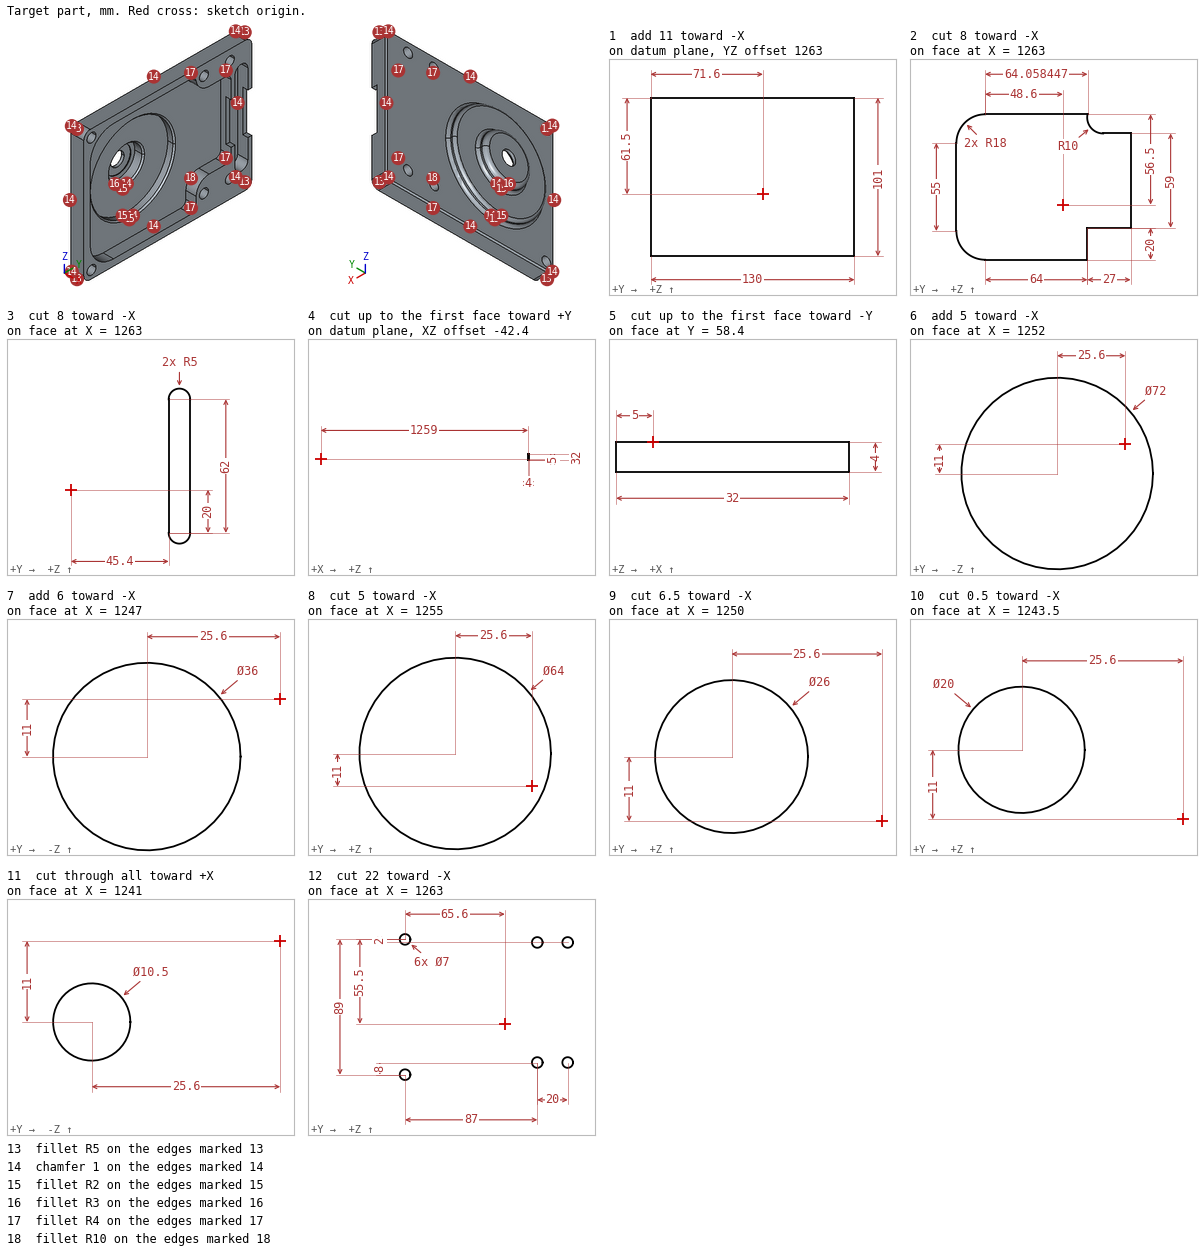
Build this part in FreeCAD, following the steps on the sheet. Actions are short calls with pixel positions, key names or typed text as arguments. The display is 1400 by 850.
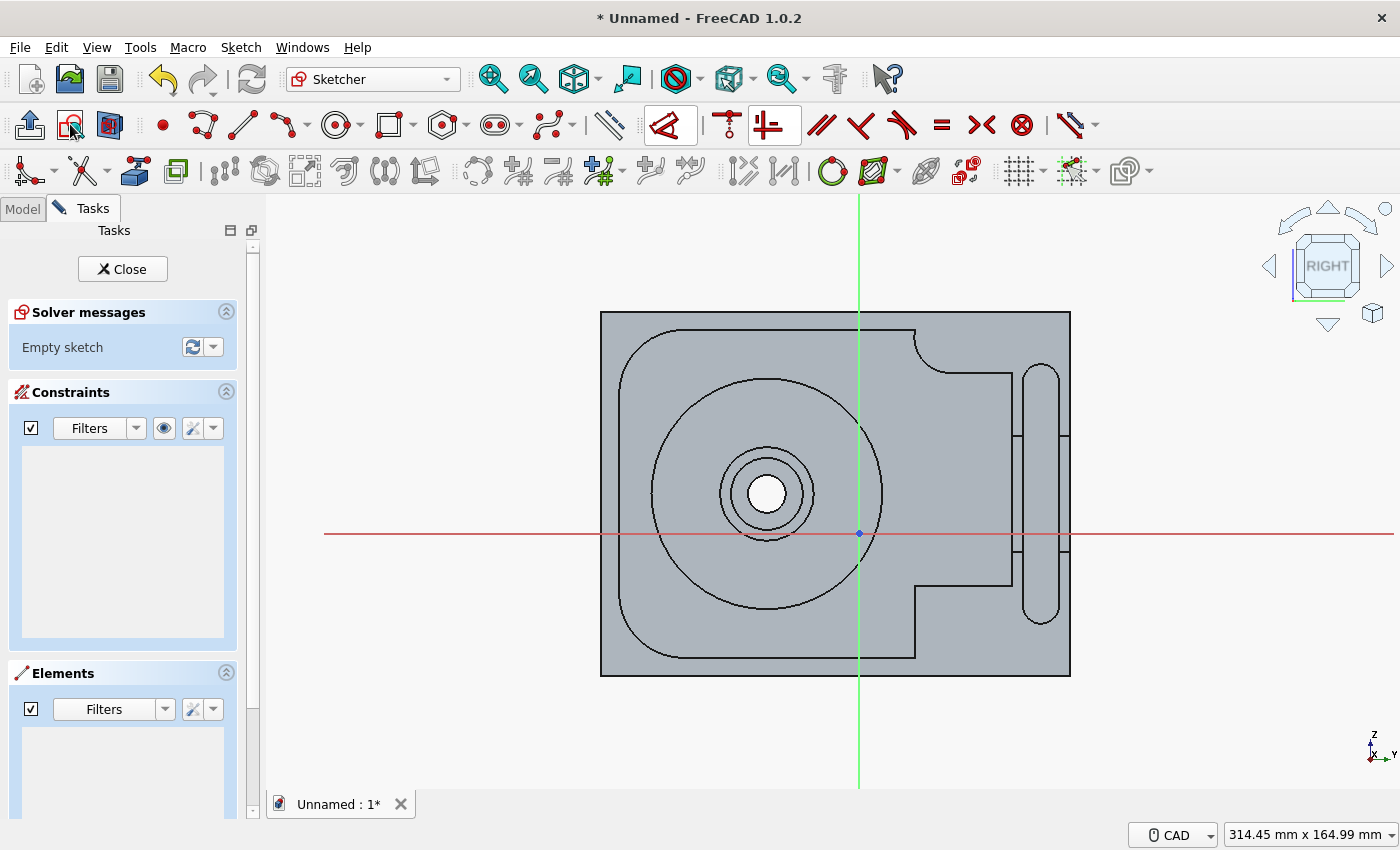
key(g)
key(c)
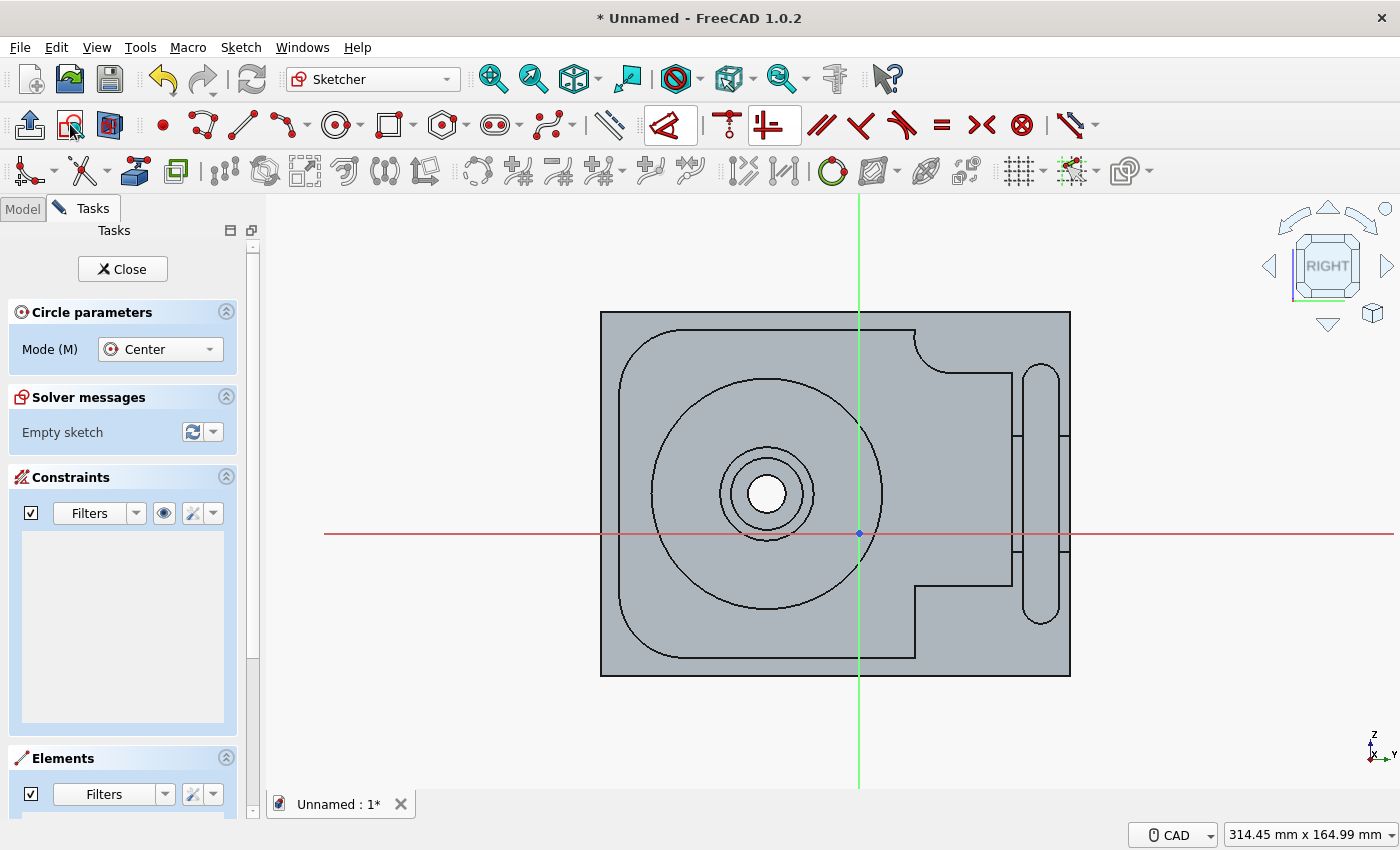
scroll(623, 333, up, 3)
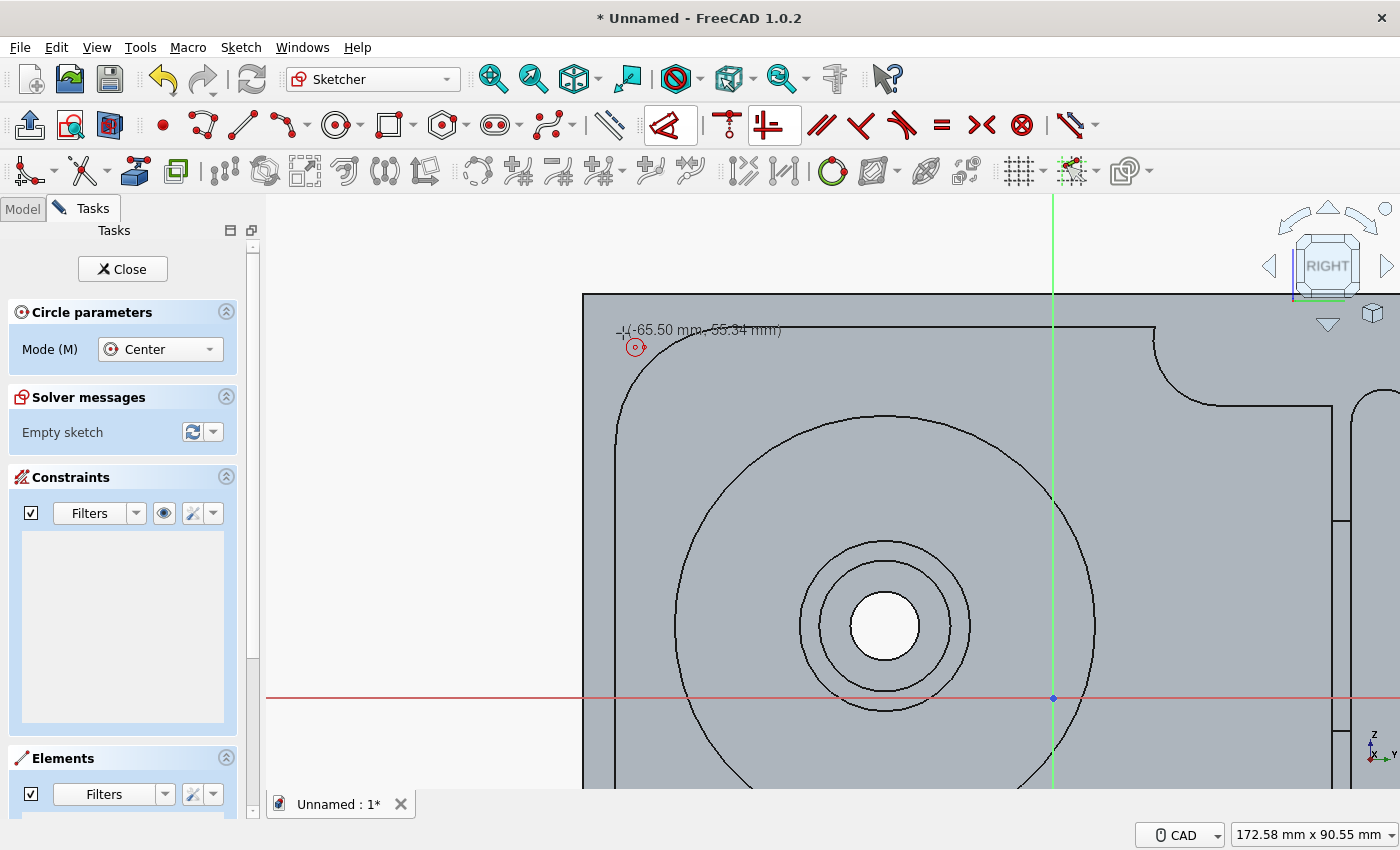
click(622, 334)
move(638, 317)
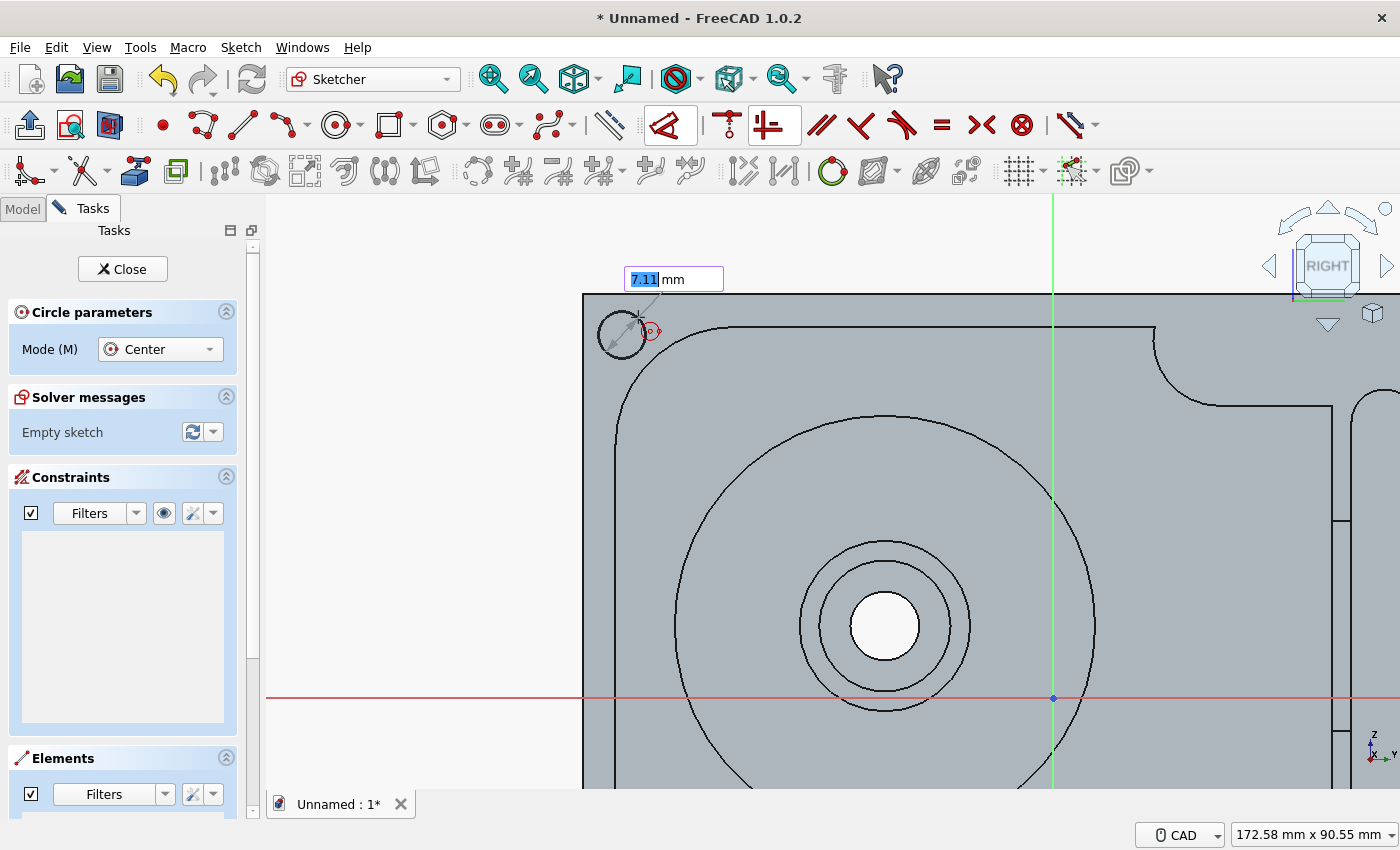
text(7)
key(Return)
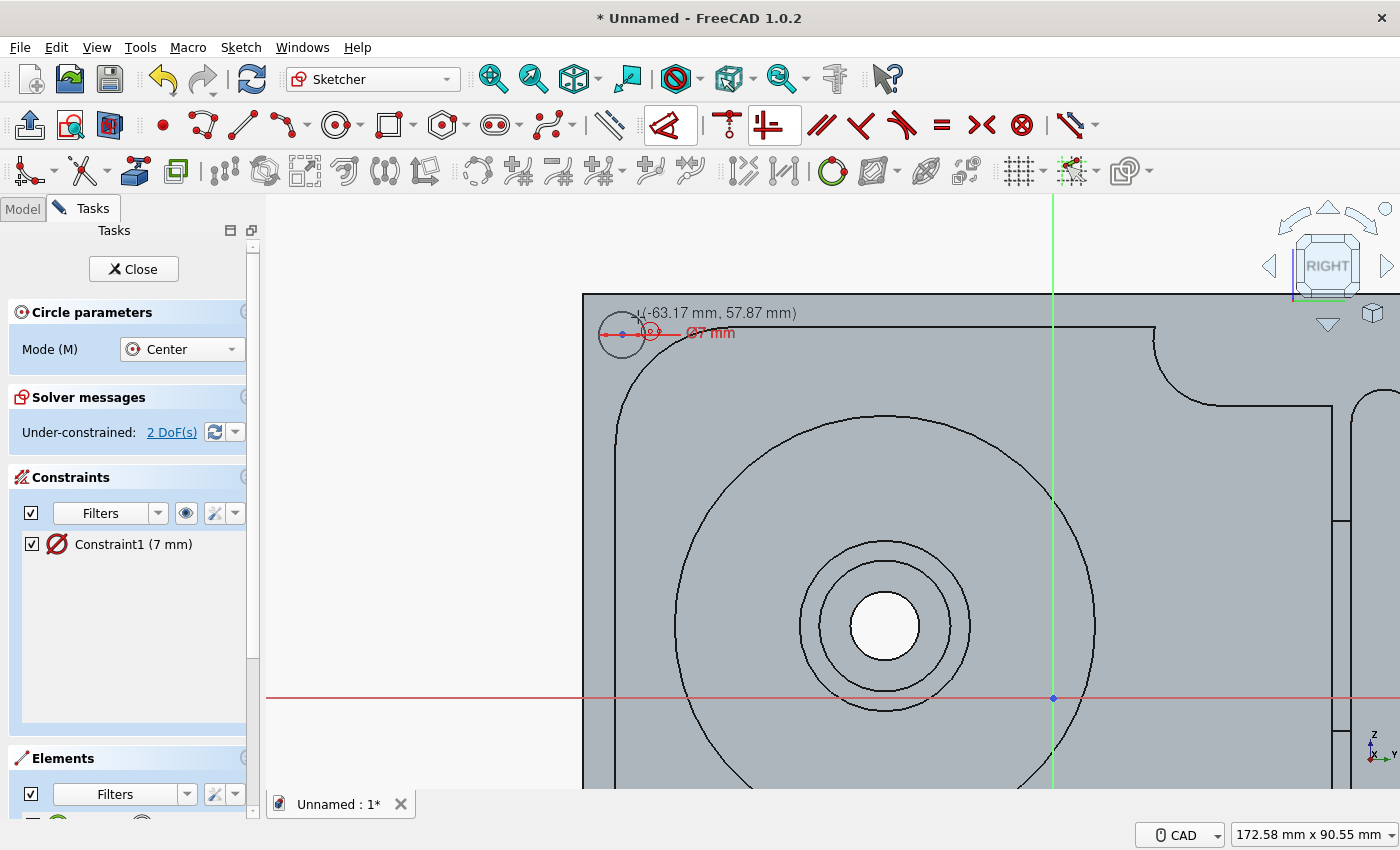
scroll(510, 328, down, 3)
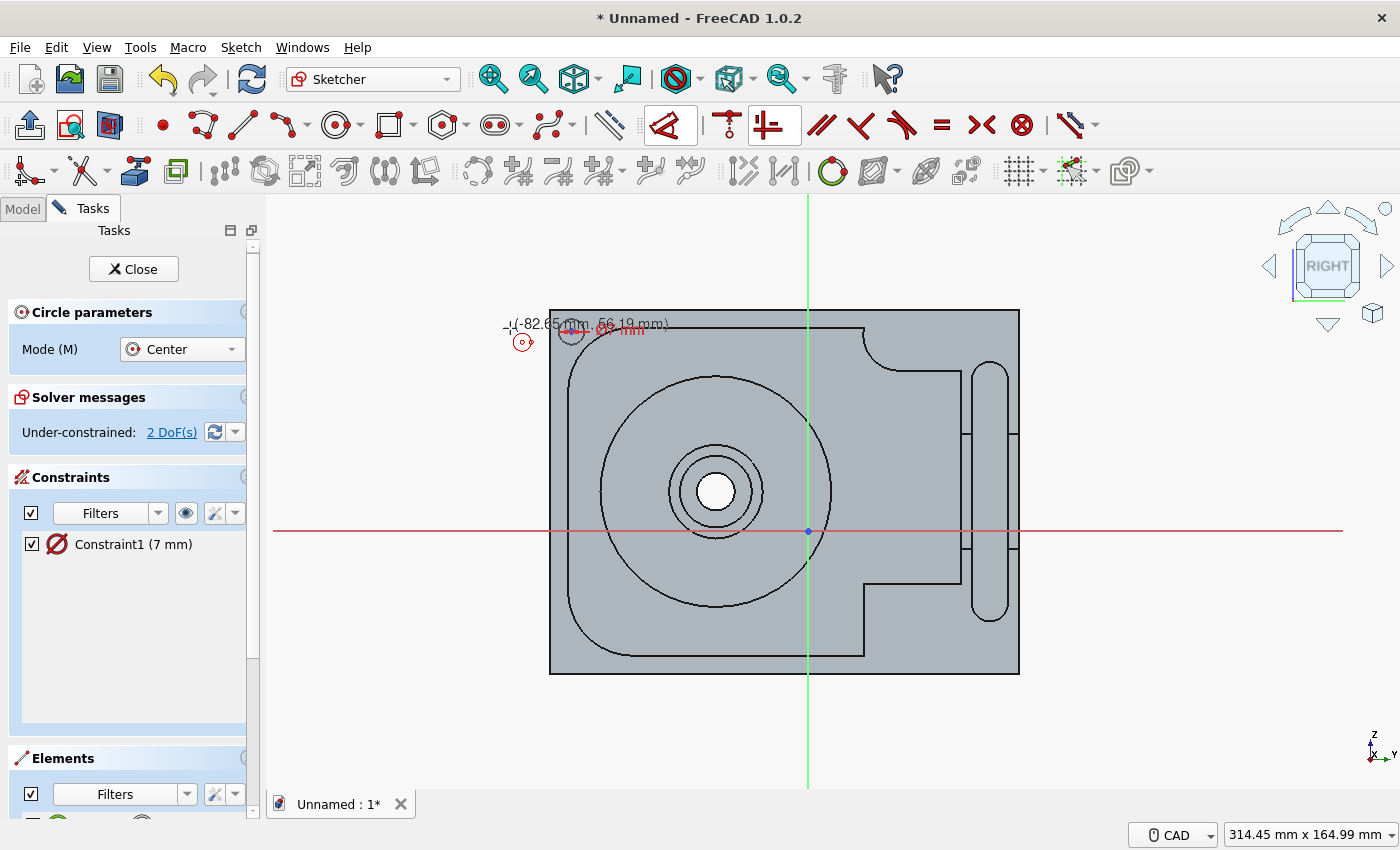
scroll(572, 652, up, 3)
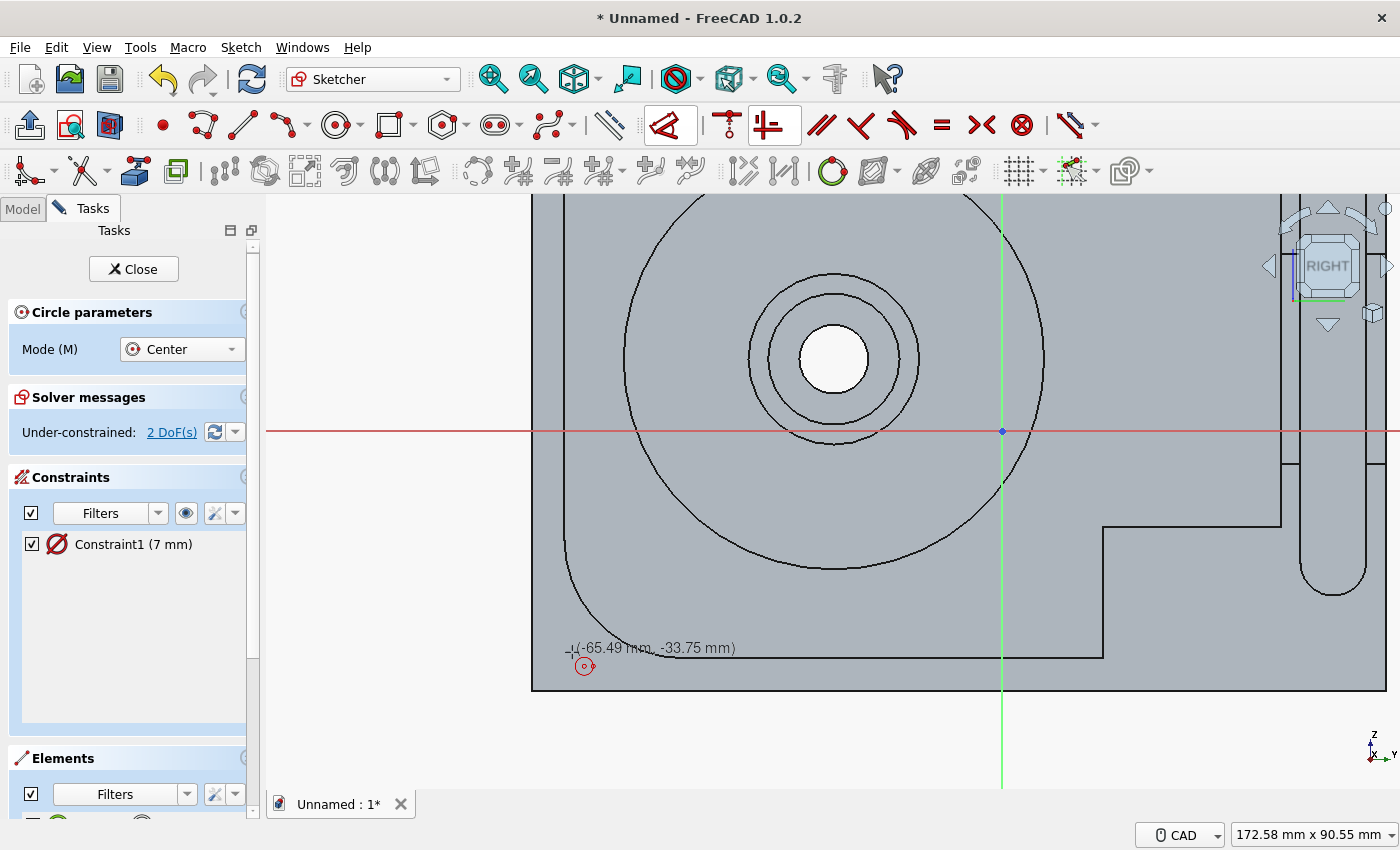
click(571, 652)
move(587, 635)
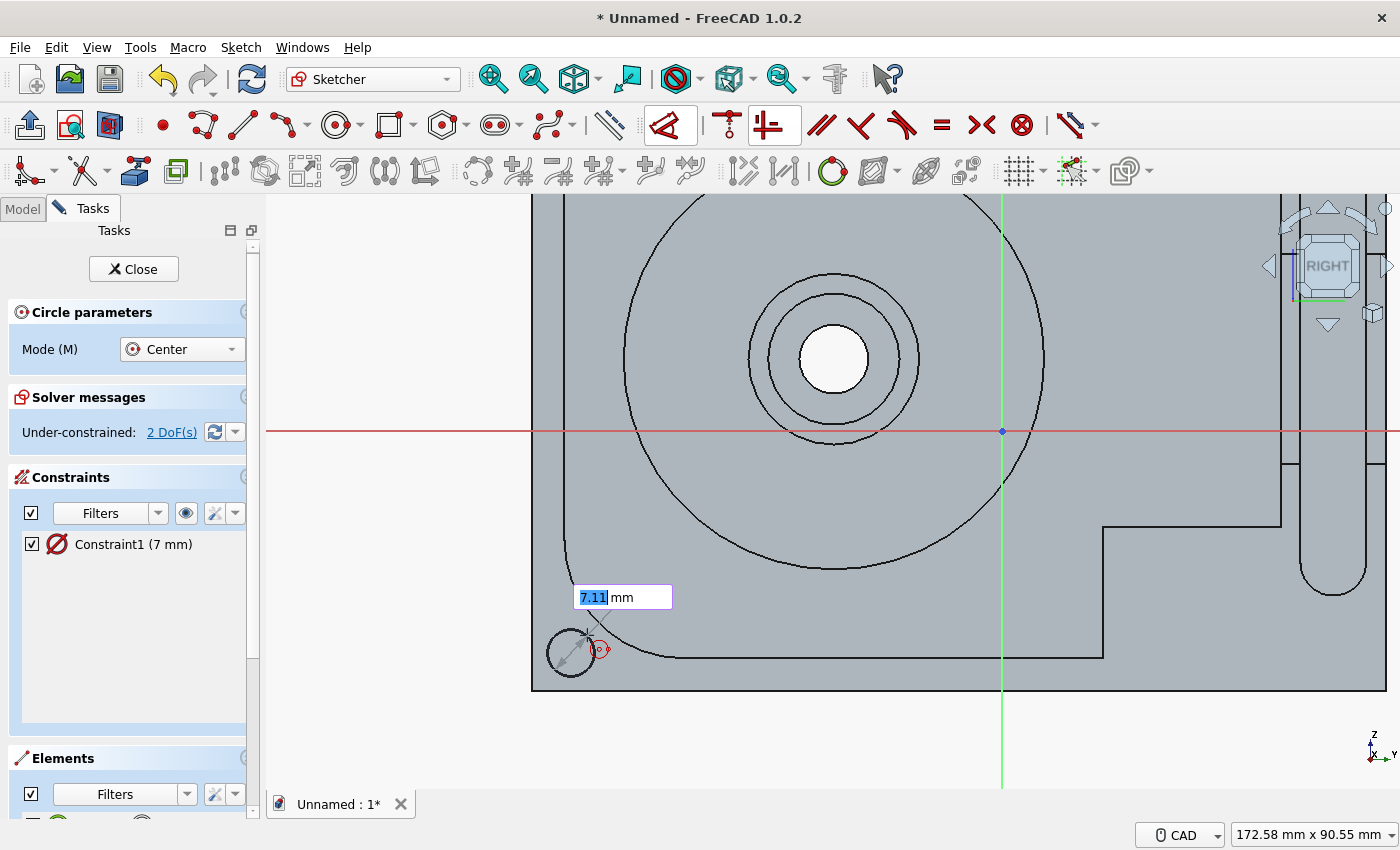
text(7)
key(Return)